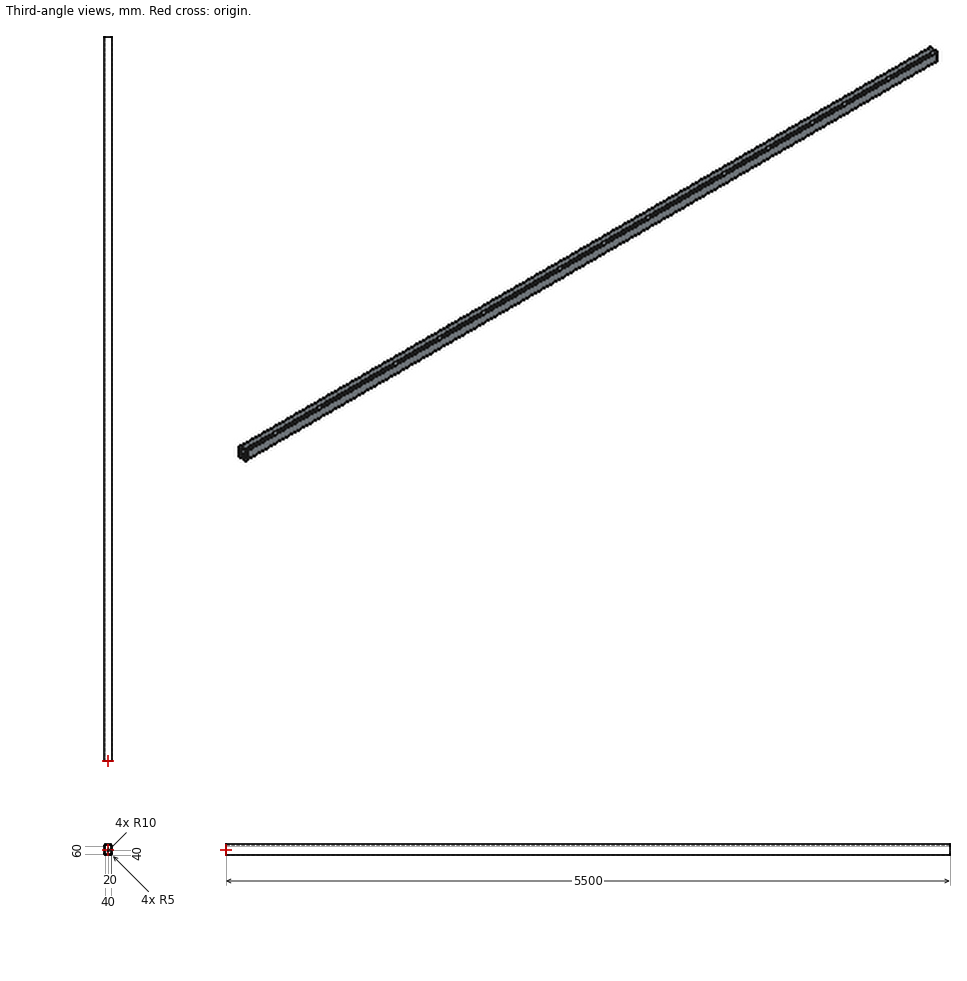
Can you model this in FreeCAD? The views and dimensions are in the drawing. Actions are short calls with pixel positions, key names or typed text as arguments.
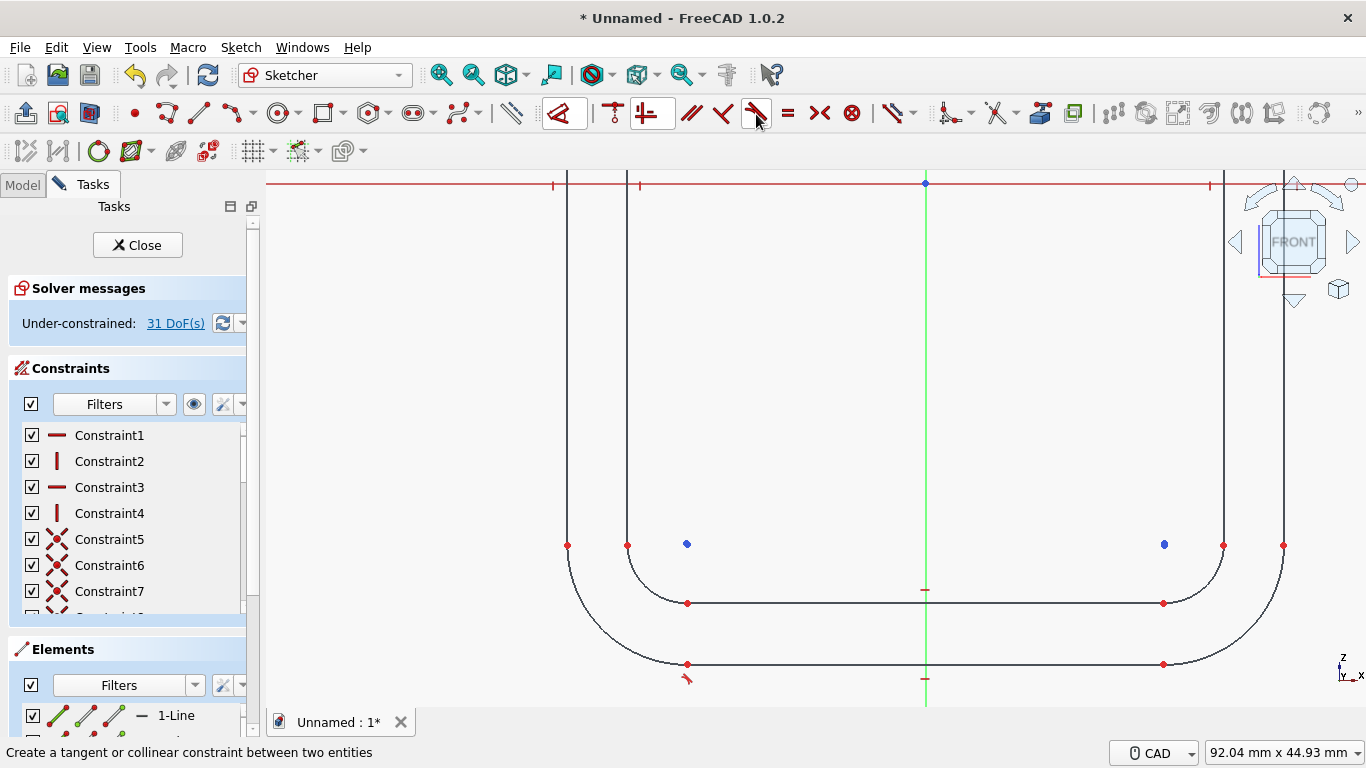
click(1021, 665)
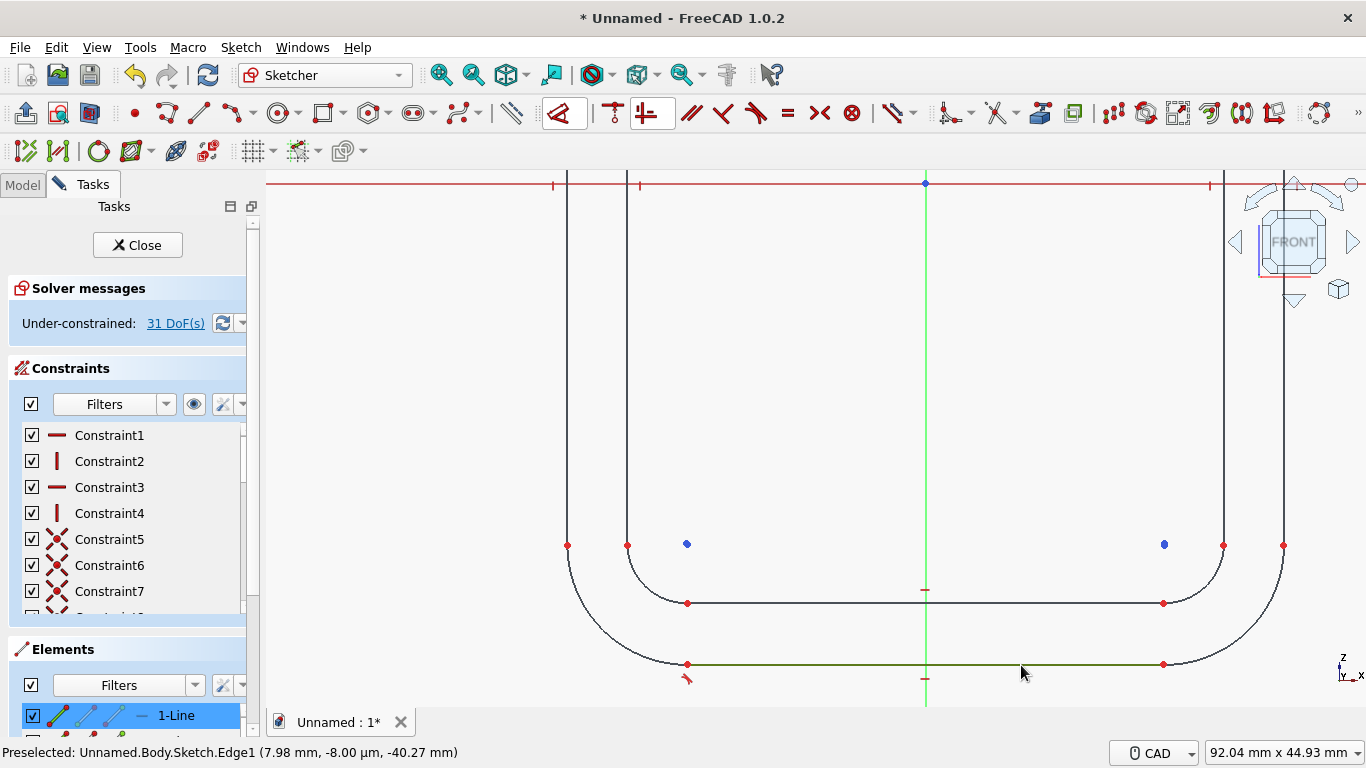
click(1201, 659)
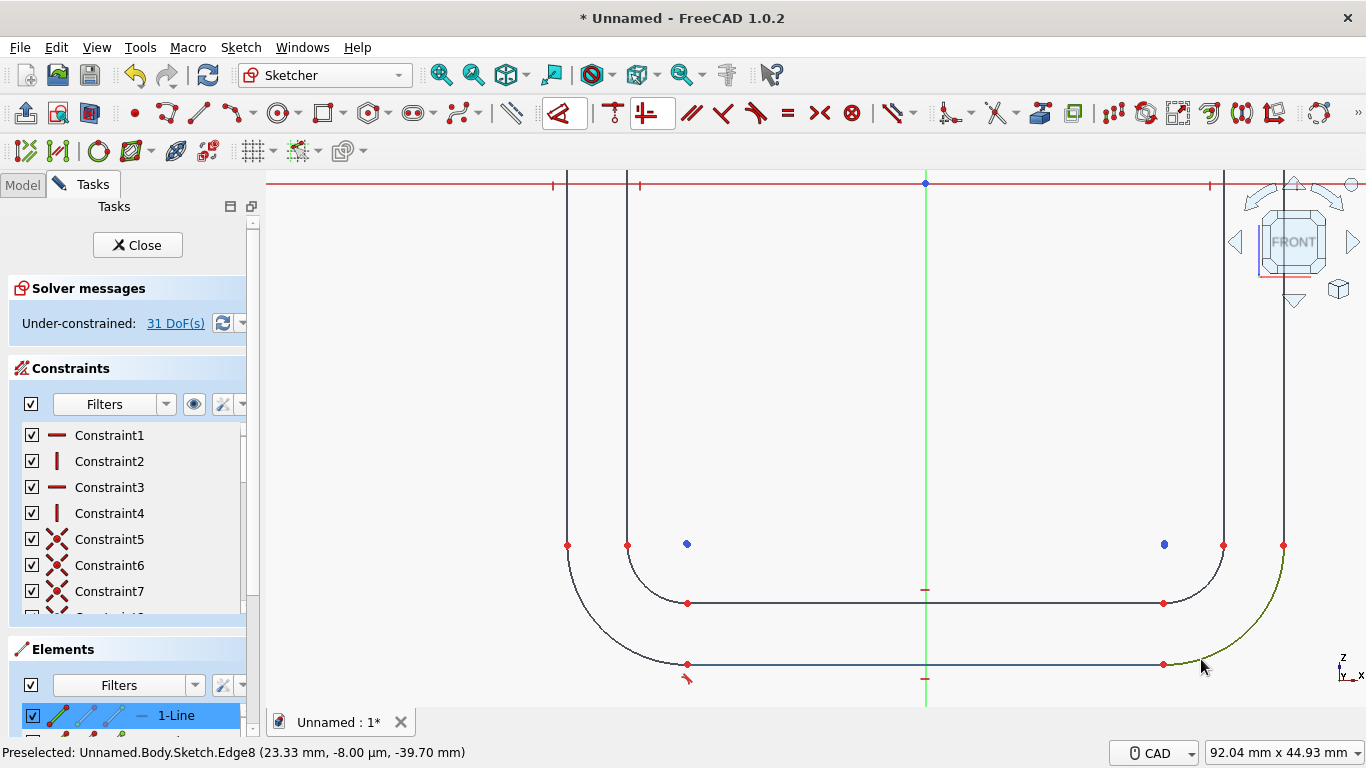
click(756, 114)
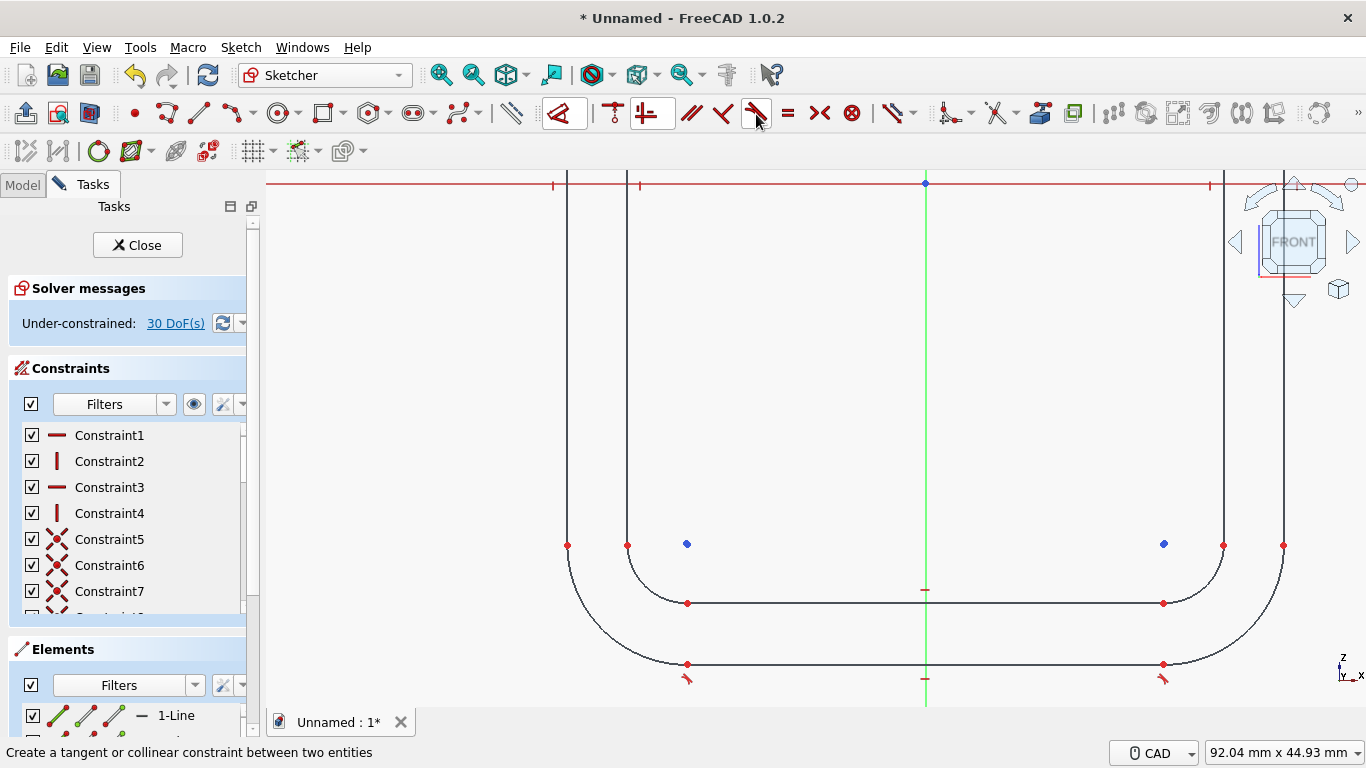
click(567, 330)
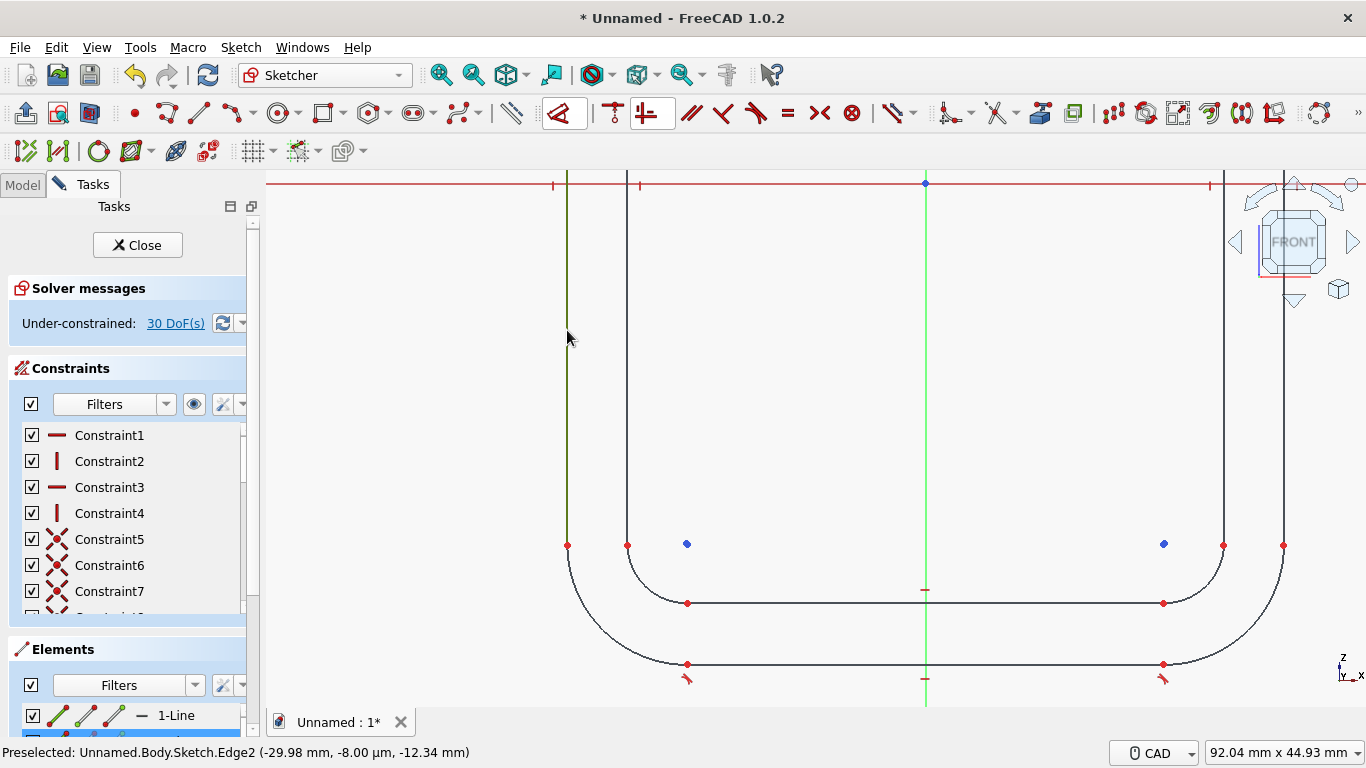
click(581, 600)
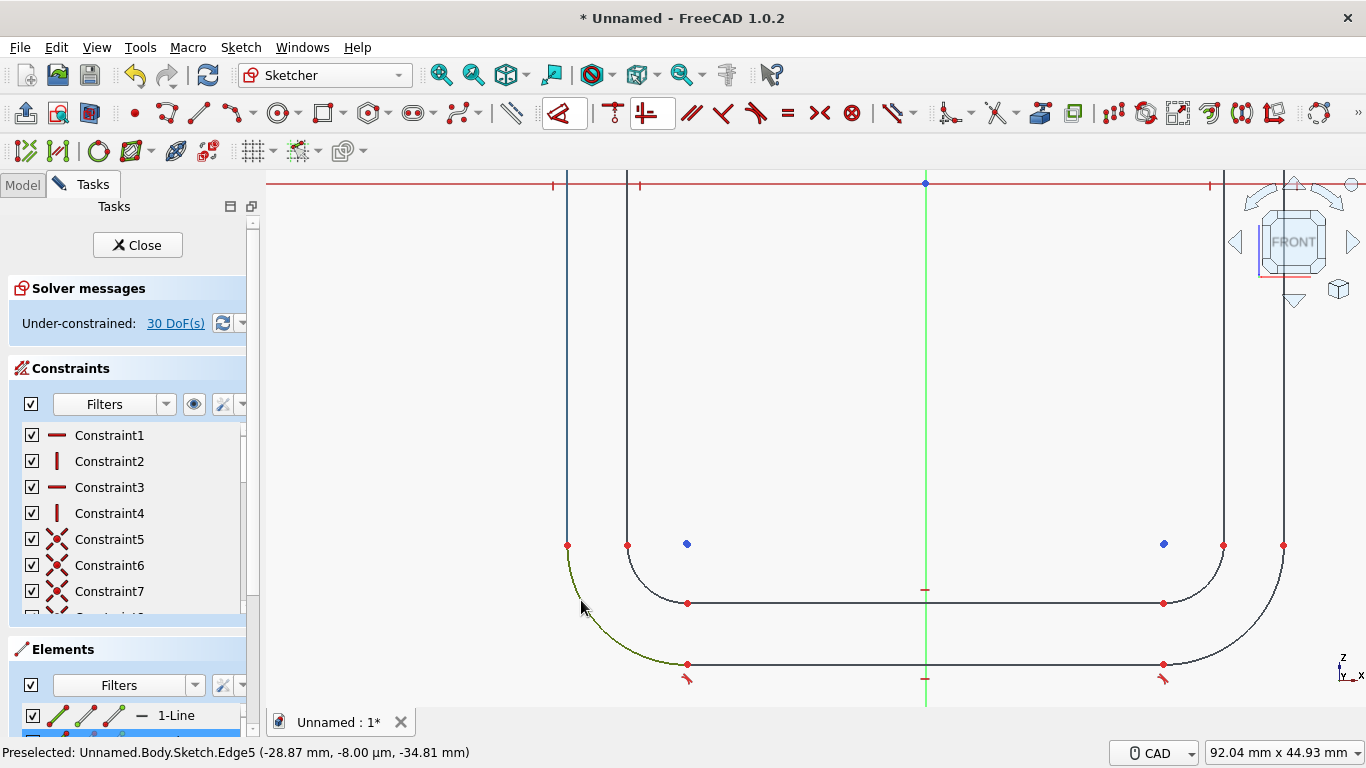
click(756, 114)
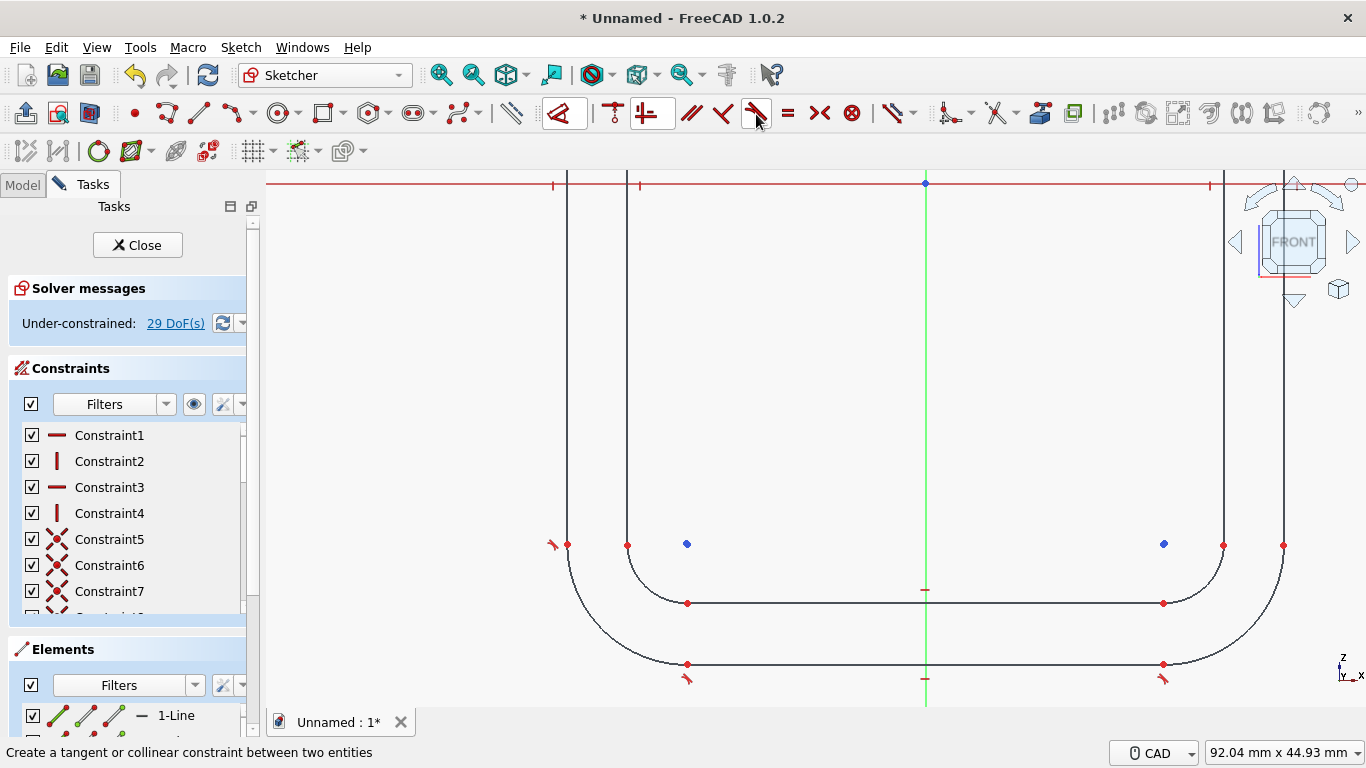
click(567, 329)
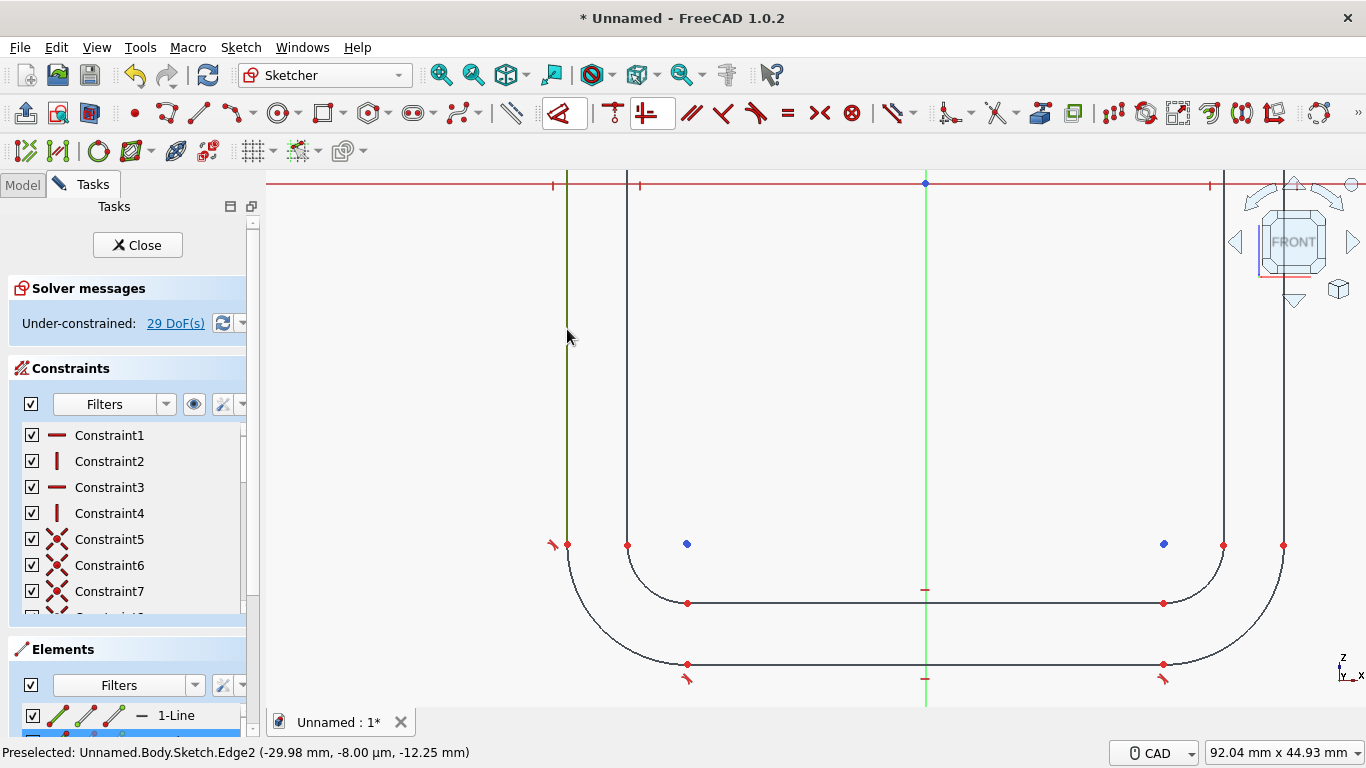
scroll(644, 587, down, 5)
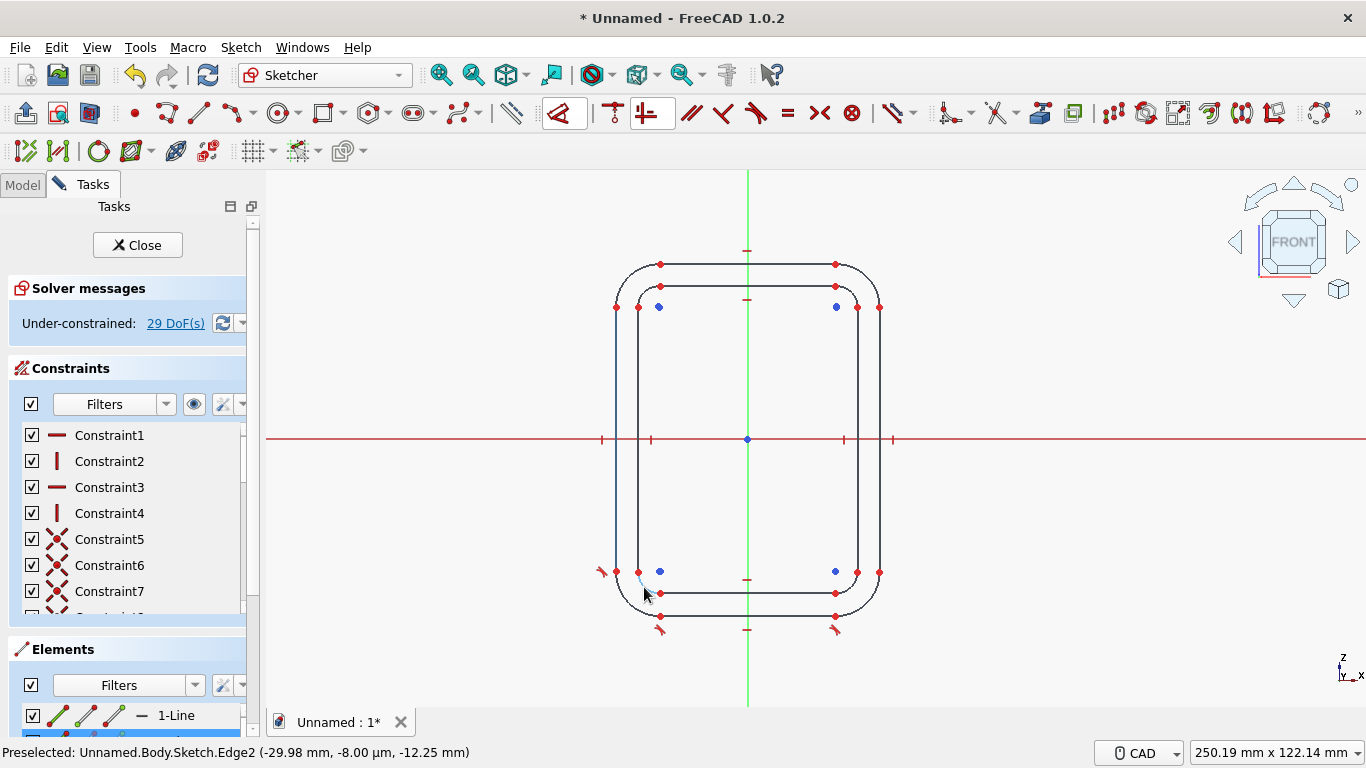
click(640, 269)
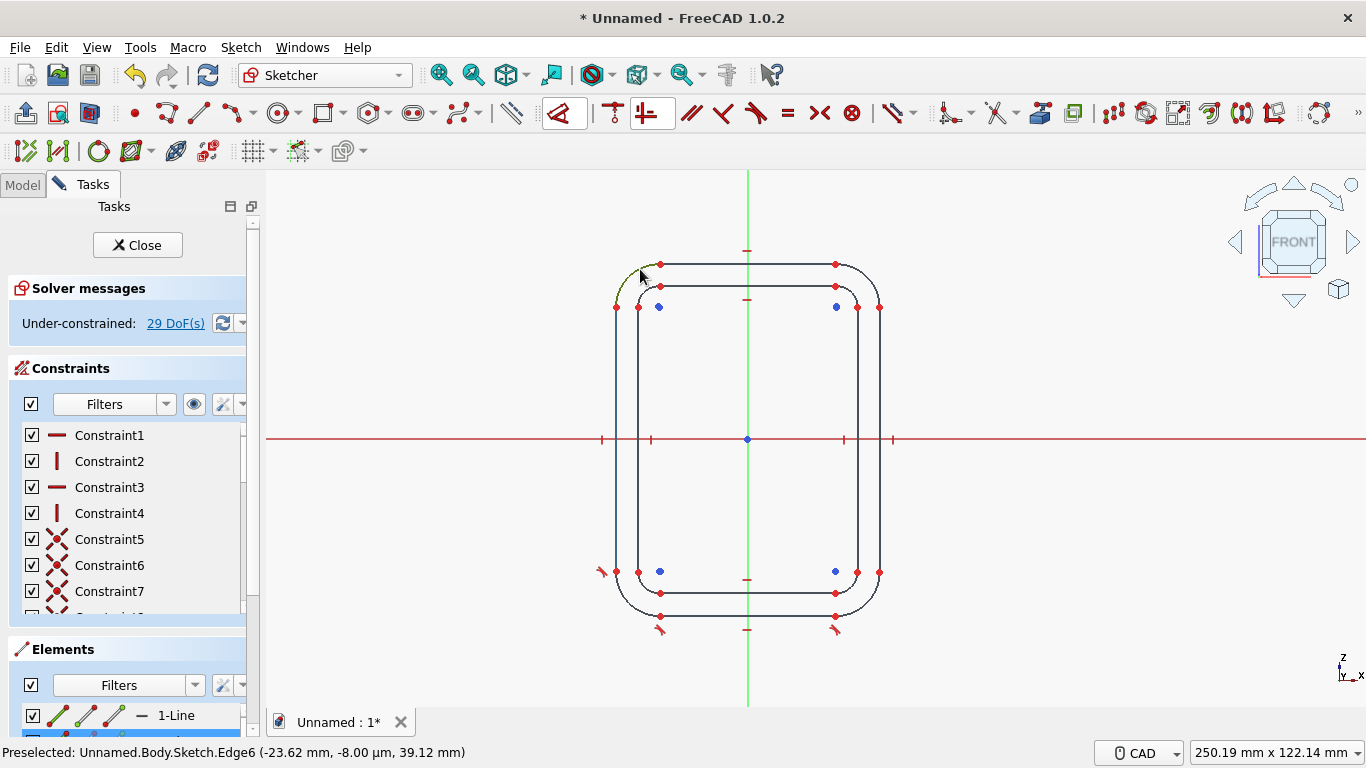
click(756, 114)